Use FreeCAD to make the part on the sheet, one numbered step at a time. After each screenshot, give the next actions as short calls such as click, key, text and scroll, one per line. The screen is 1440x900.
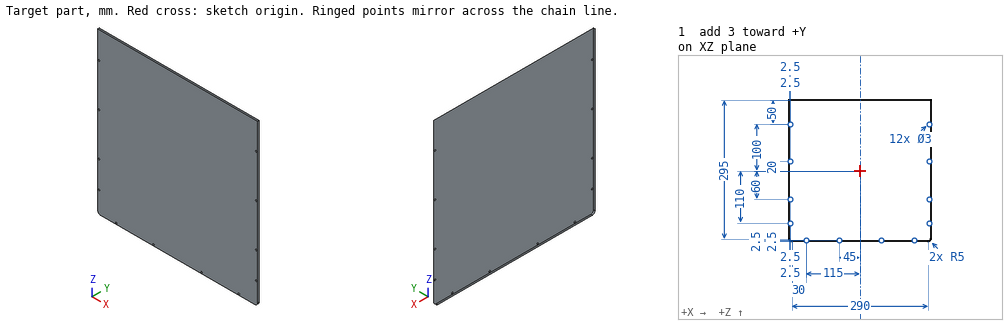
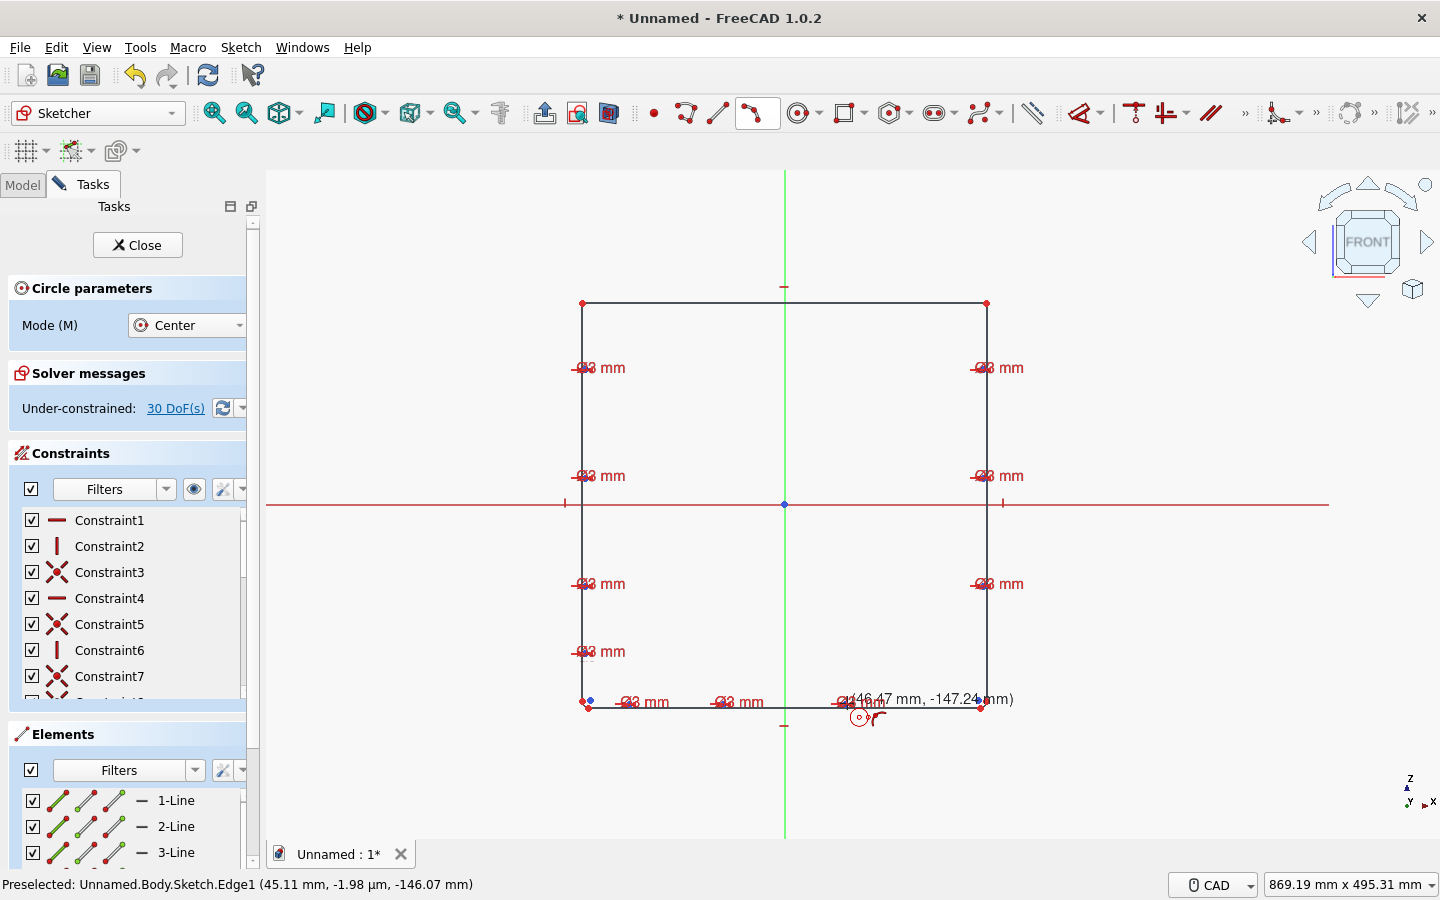
scroll(984, 654, up, 13)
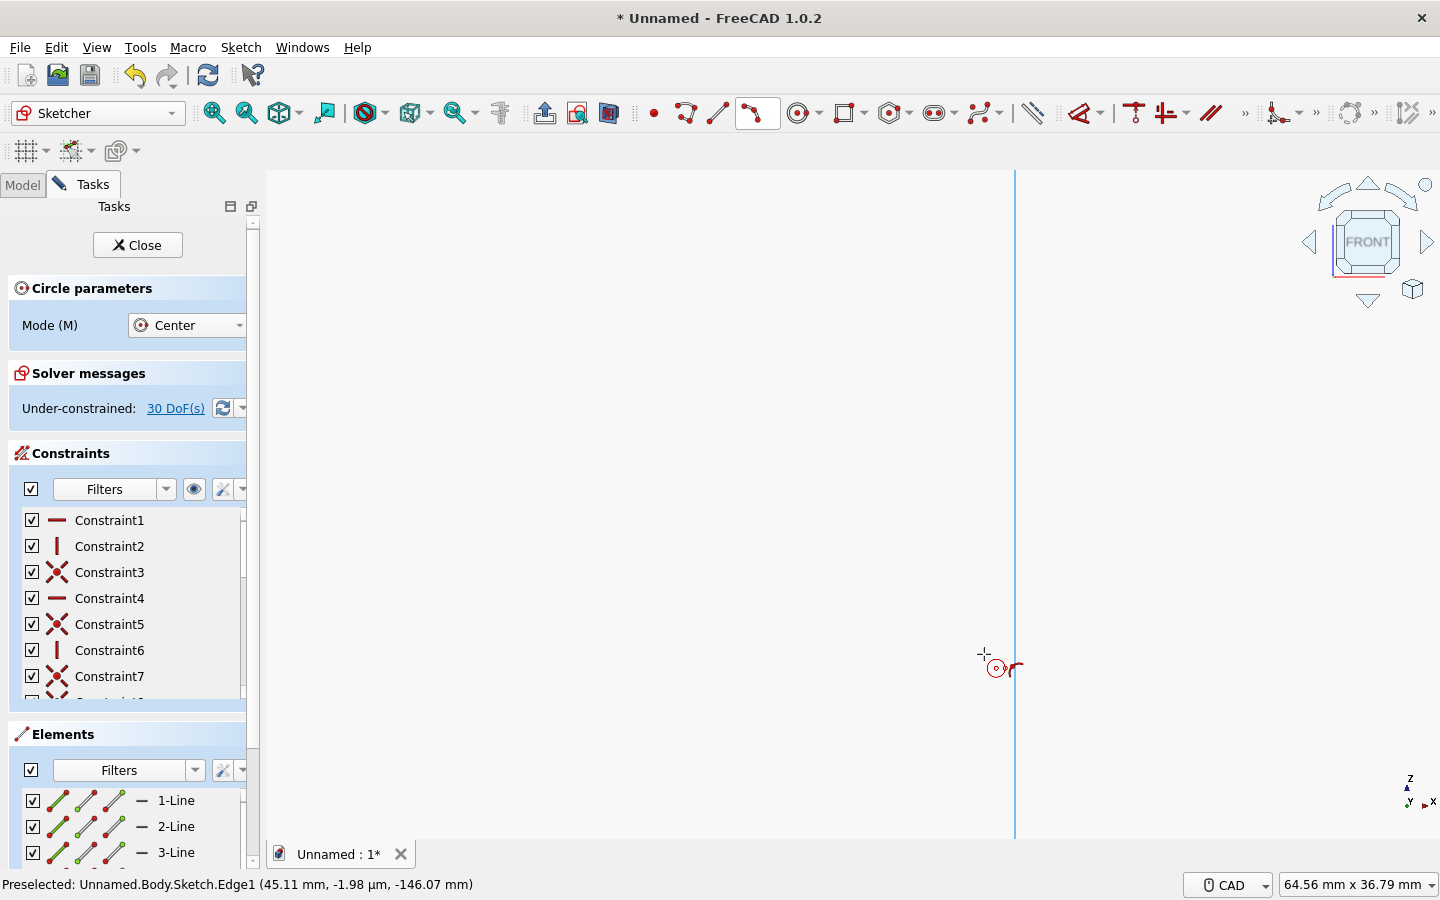
click(974, 639)
move(993, 620)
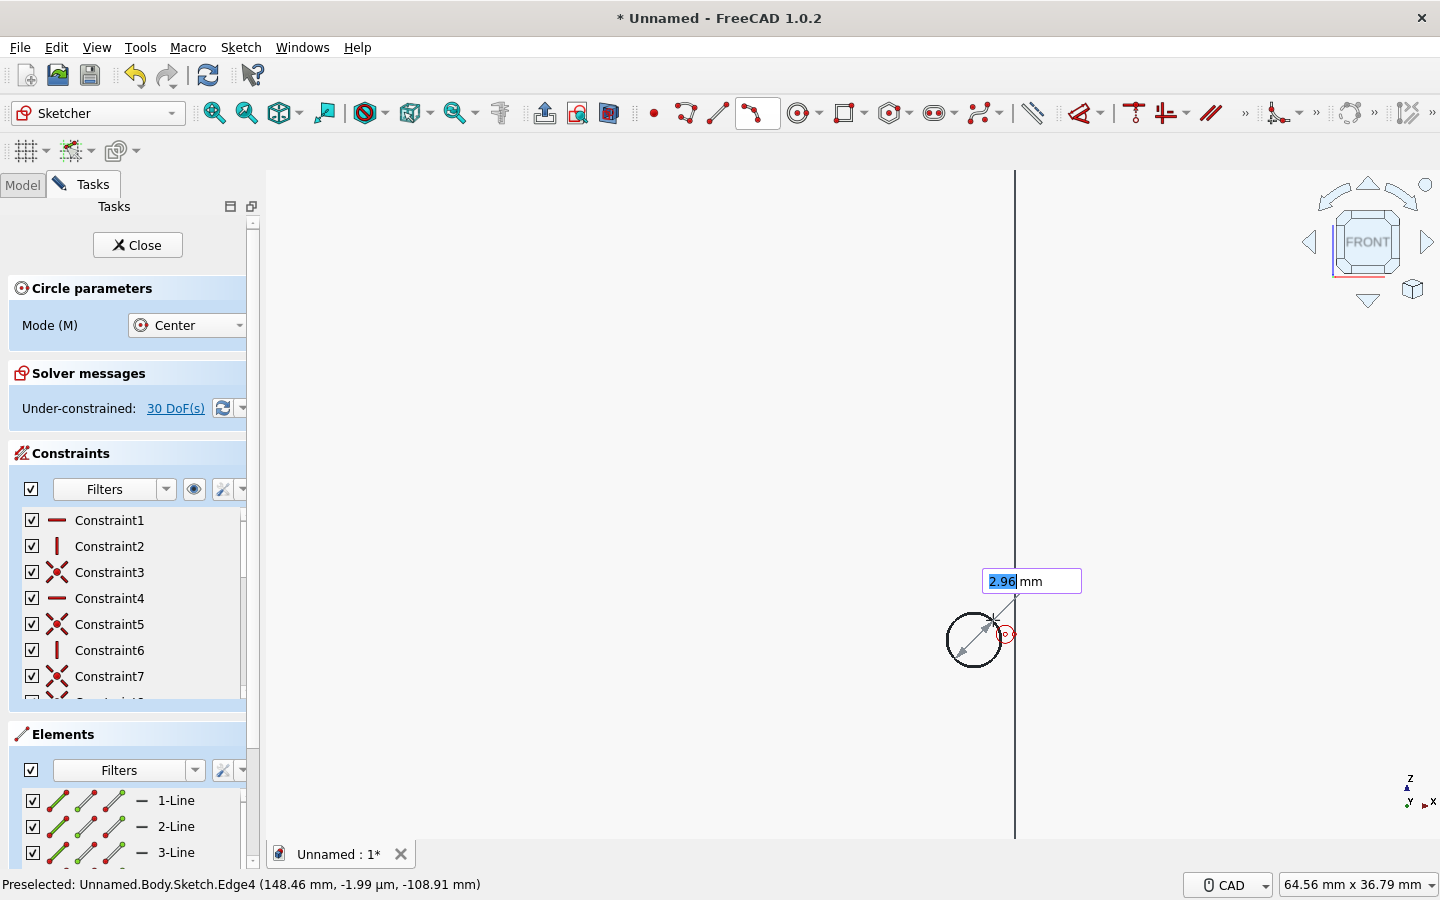
text(3)
key(Return)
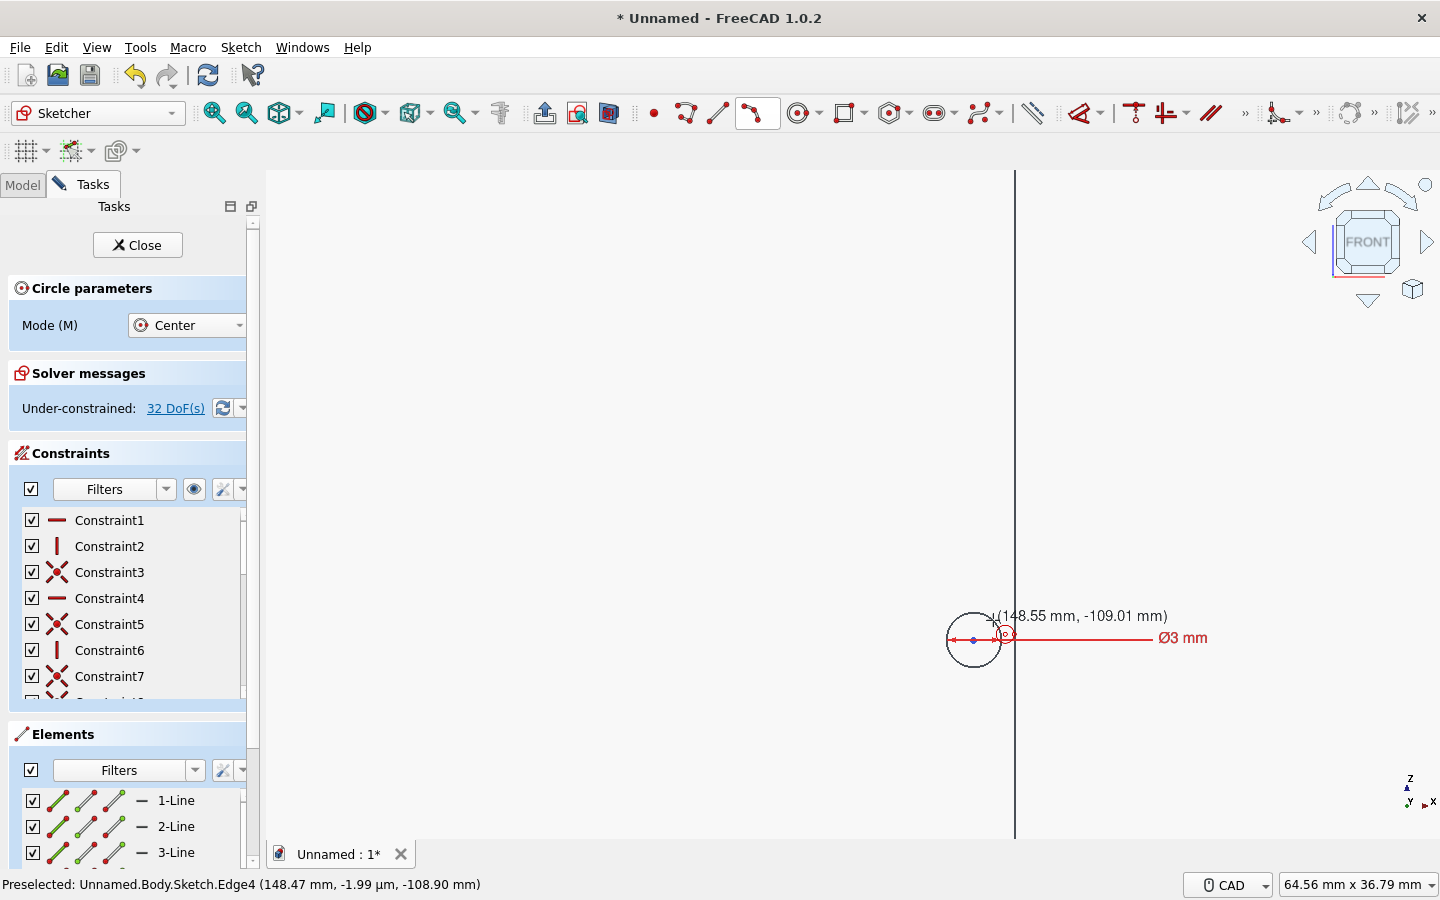
scroll(985, 654, down, 13)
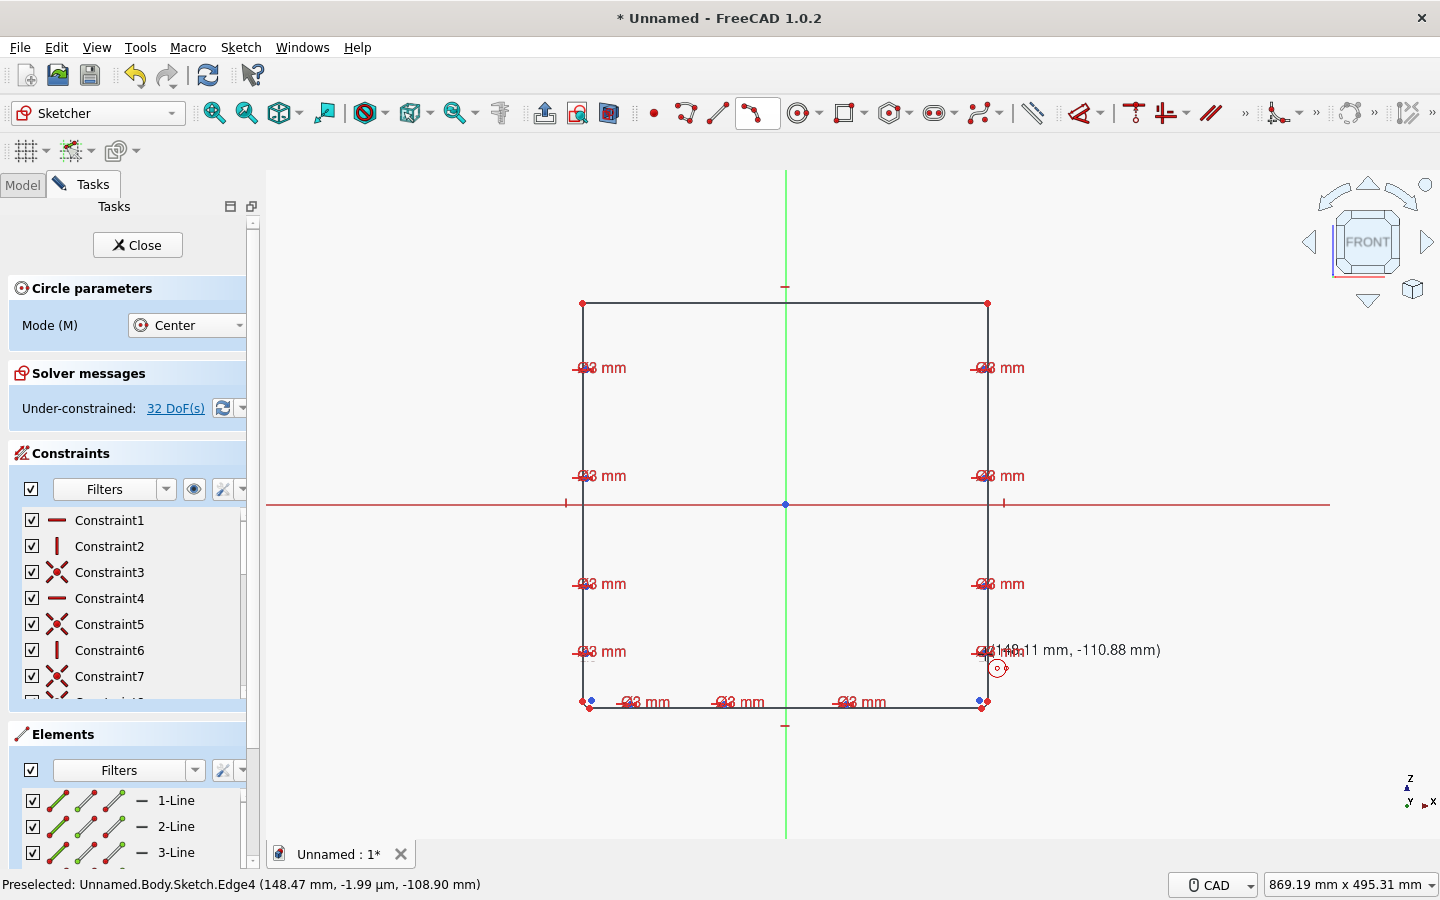
scroll(941, 704, up, 13)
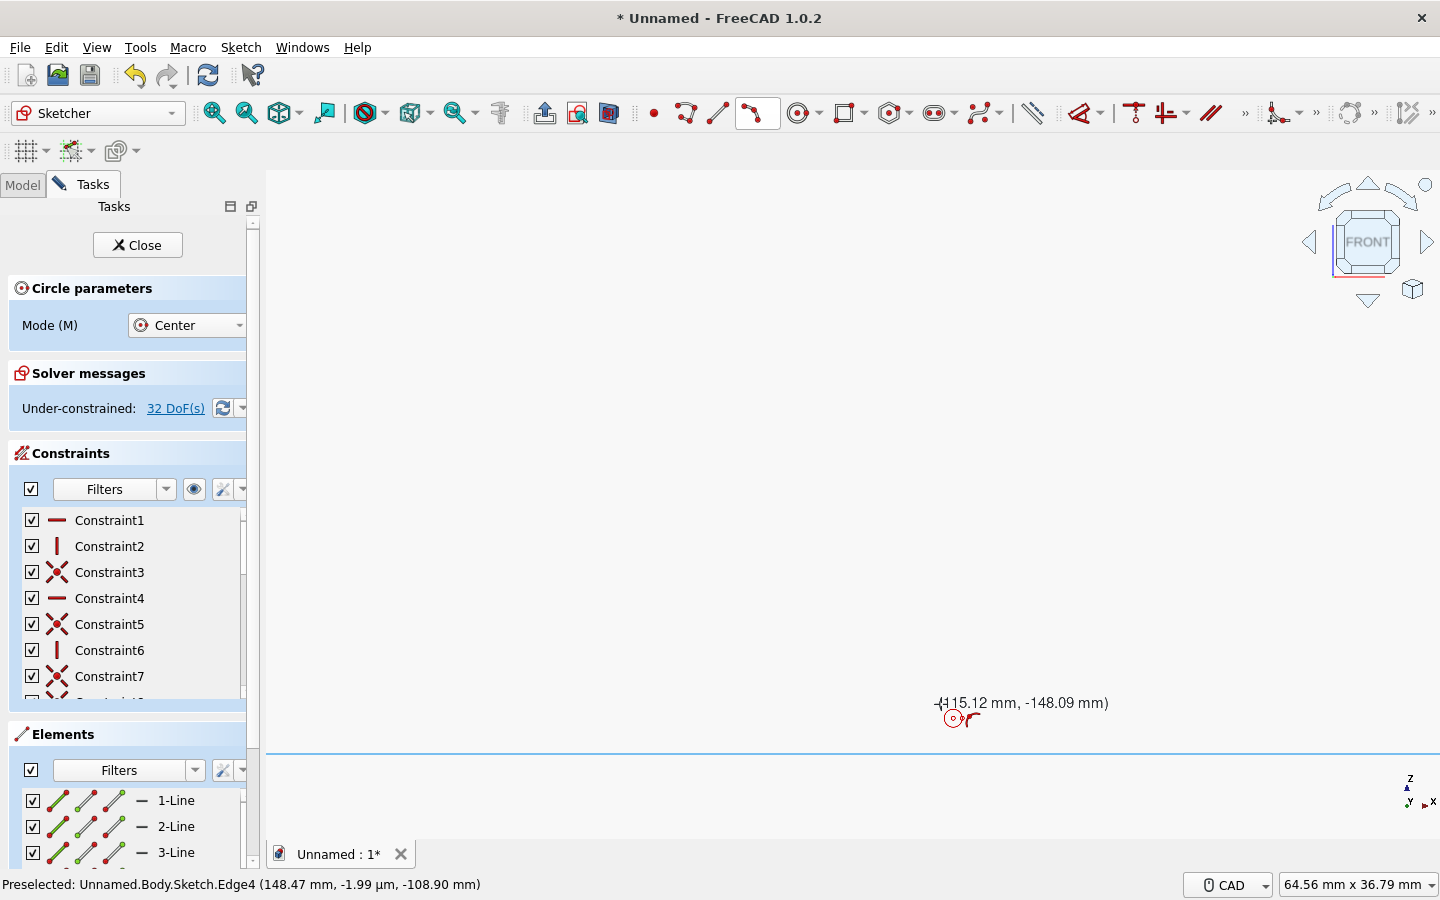
click(932, 697)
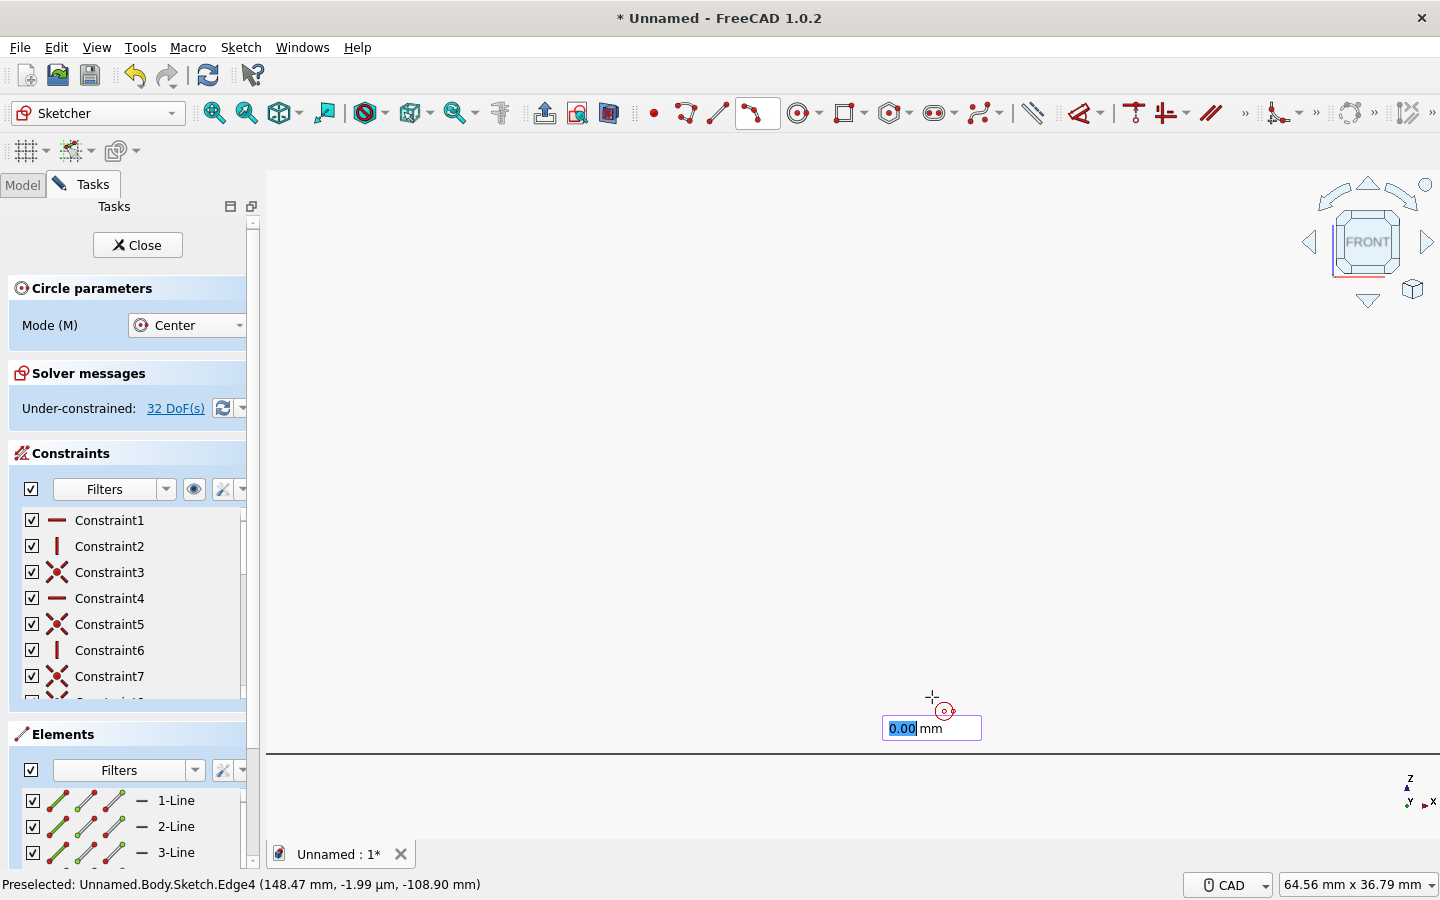
scroll(940, 704, down, 13)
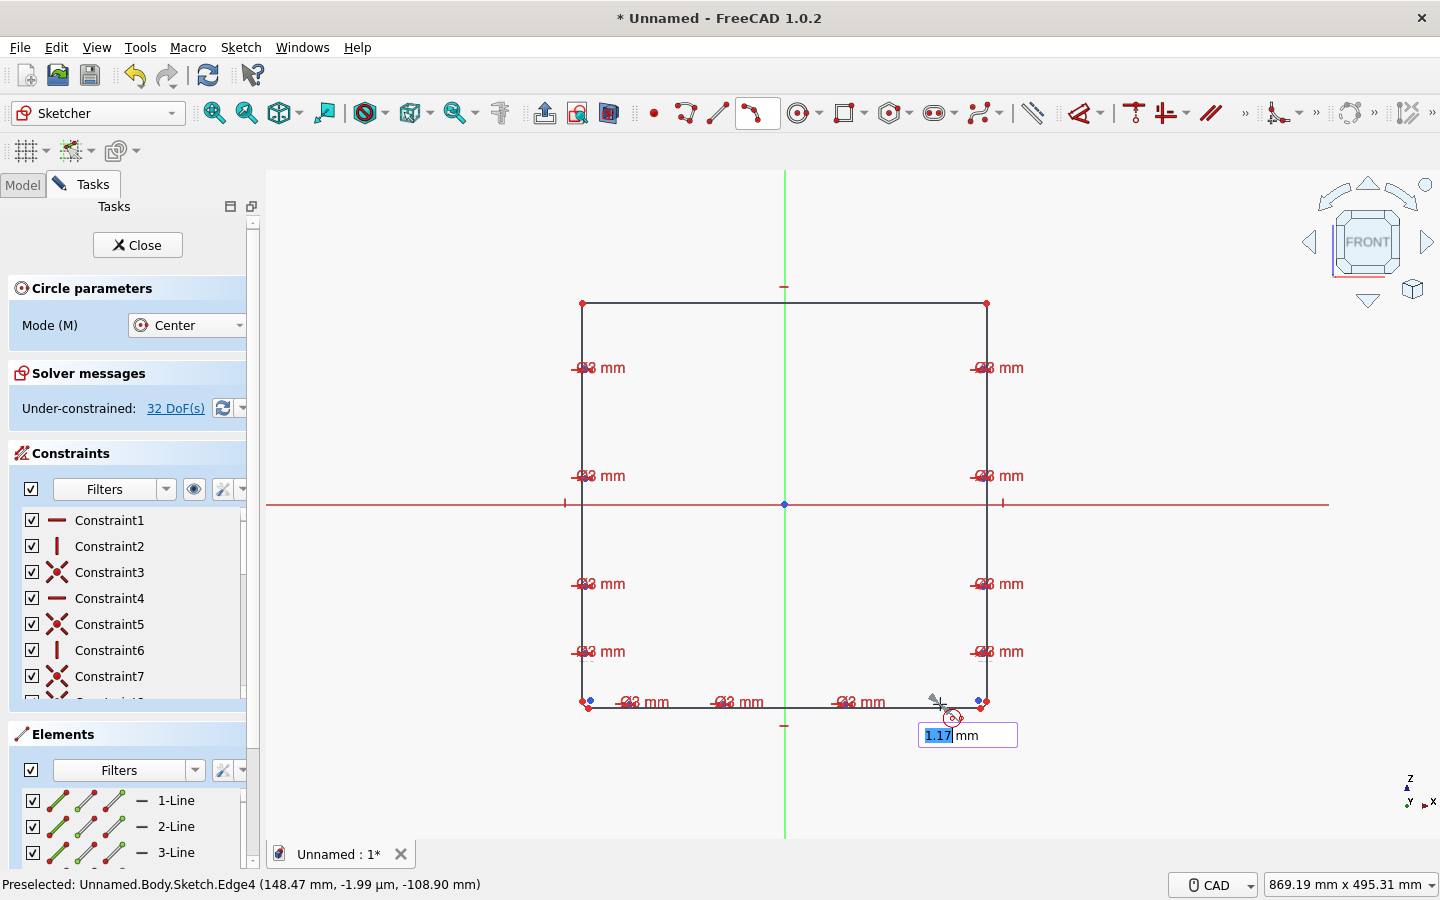
scroll(941, 703, up, 6)
move(941, 700)